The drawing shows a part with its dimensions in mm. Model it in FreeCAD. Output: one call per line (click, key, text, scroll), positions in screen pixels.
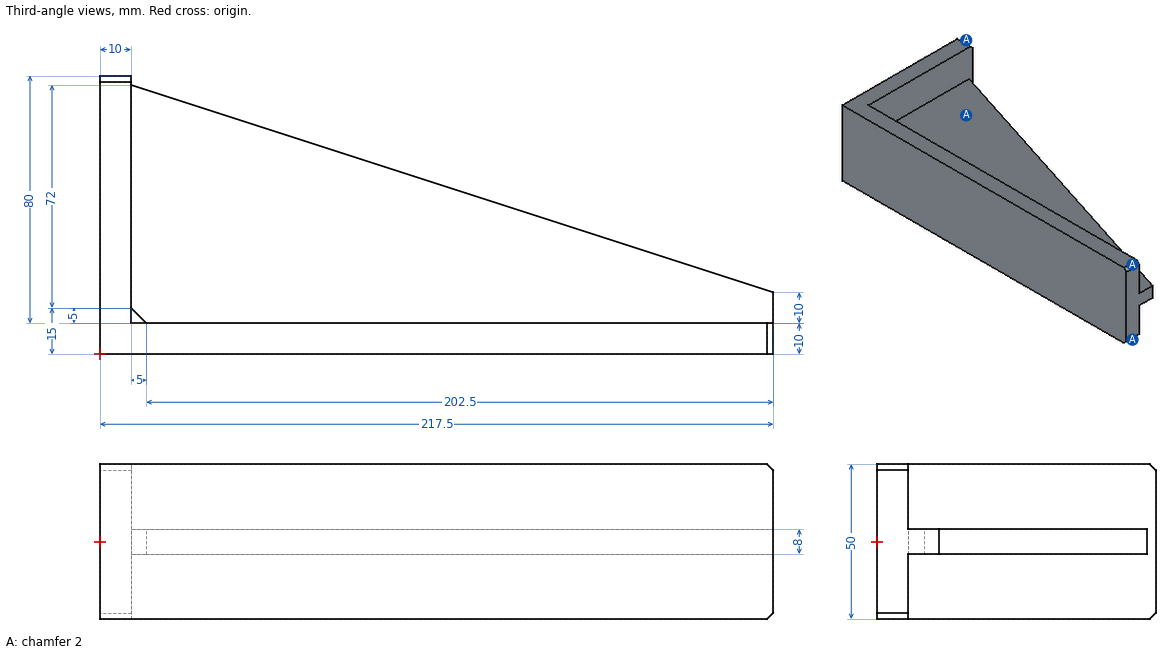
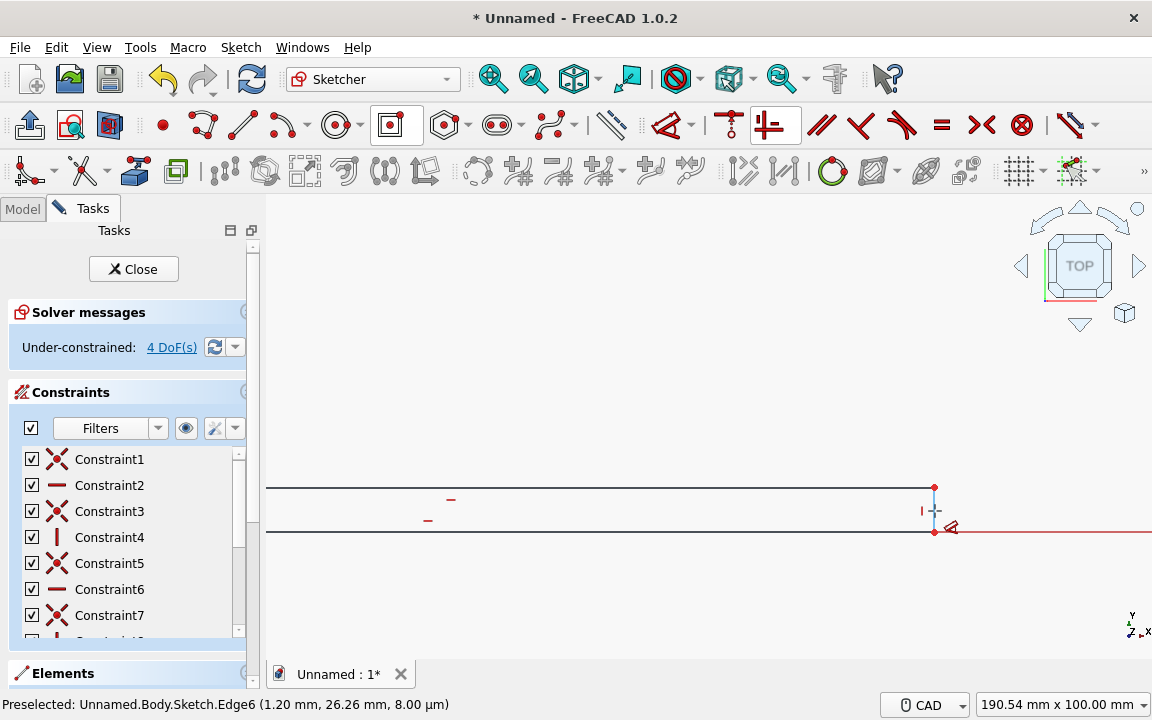
click(934, 510)
click(968, 510)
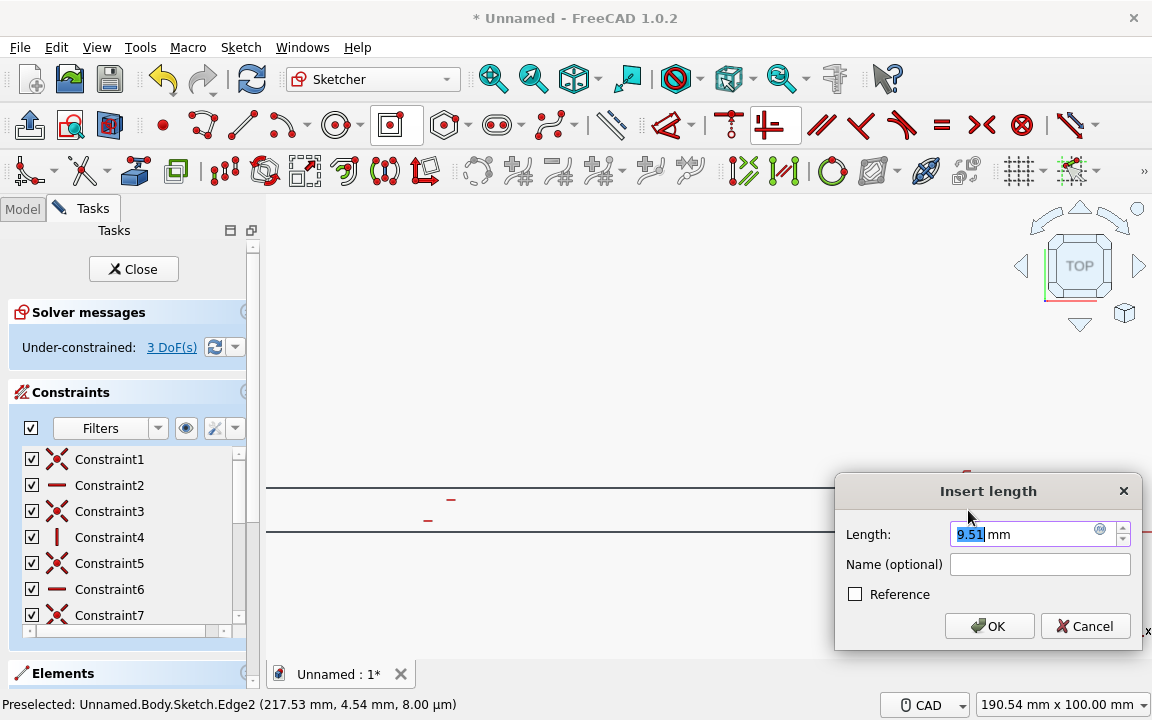
text(10)
key(Return)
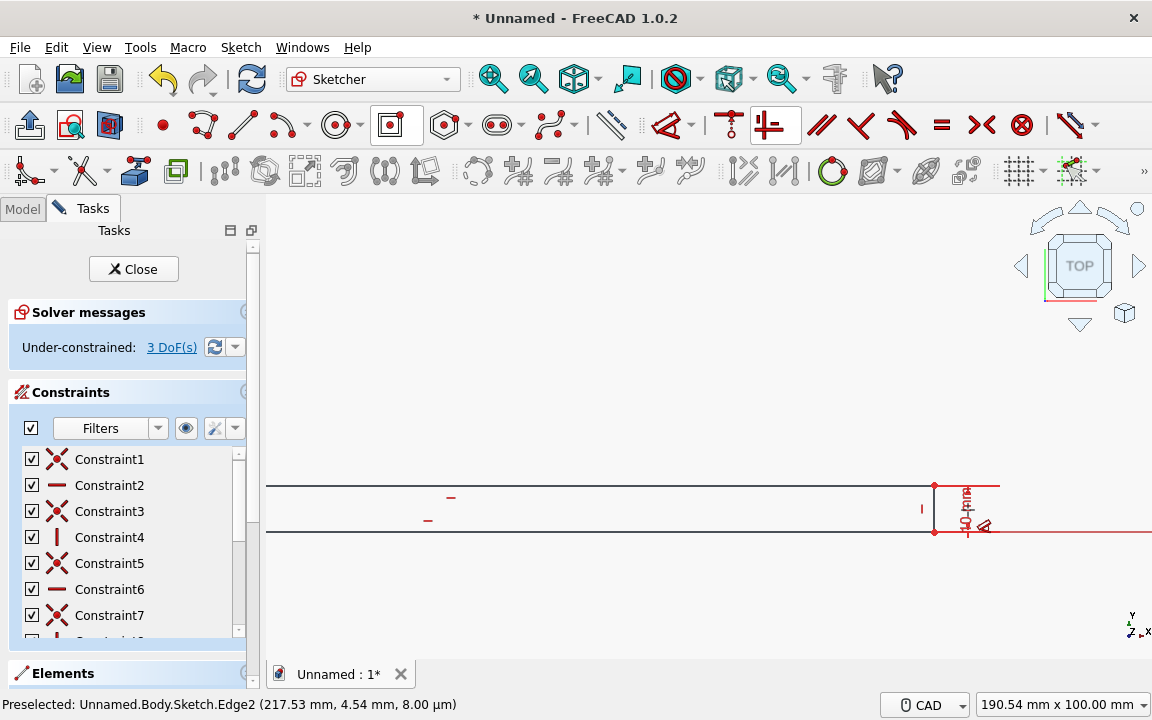
scroll(814, 511, down, 4)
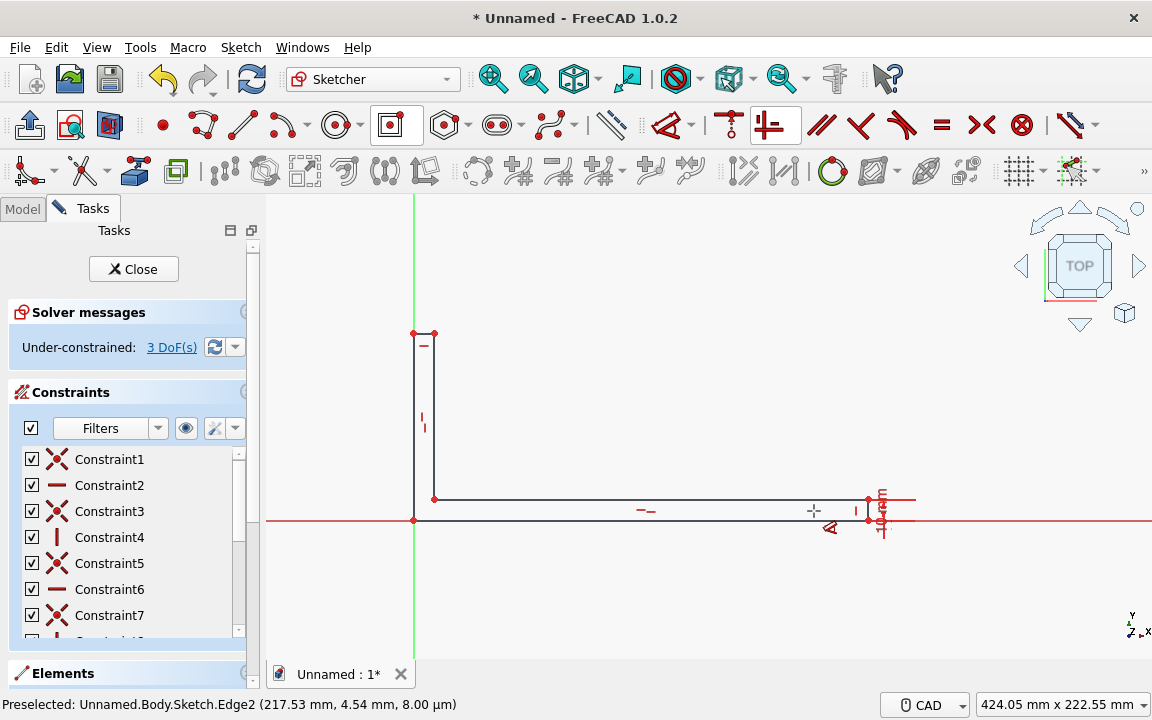
click(434, 450)
click(400, 417)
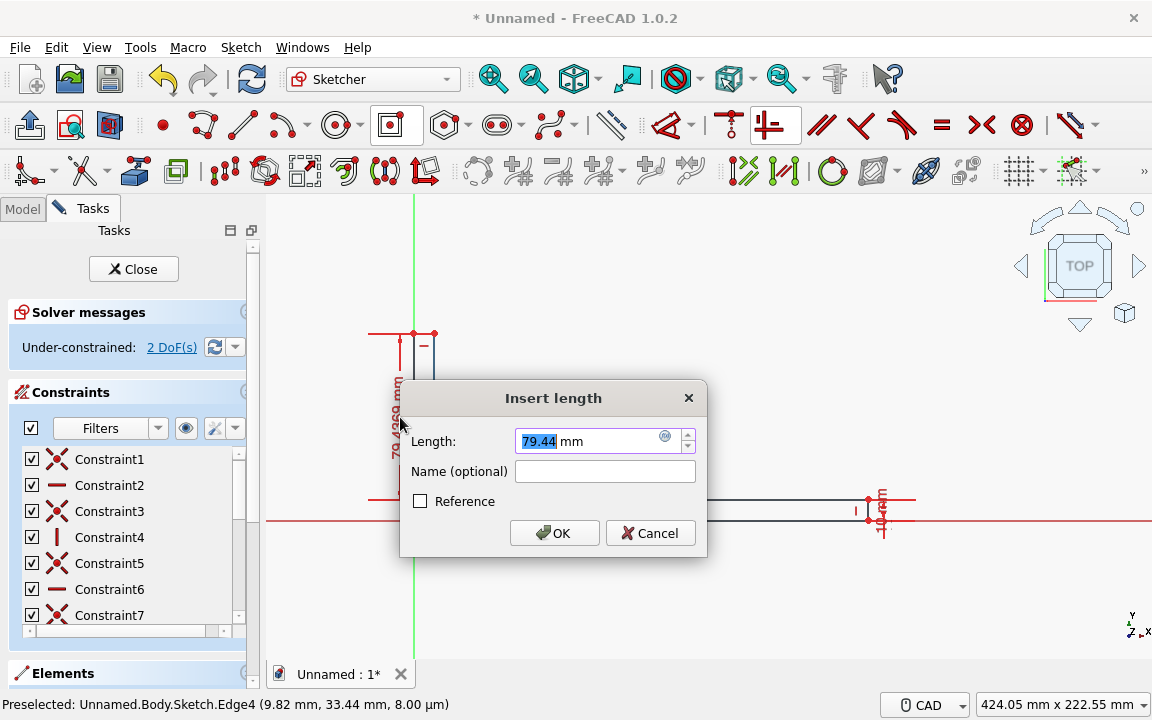
text(80)
key(Return)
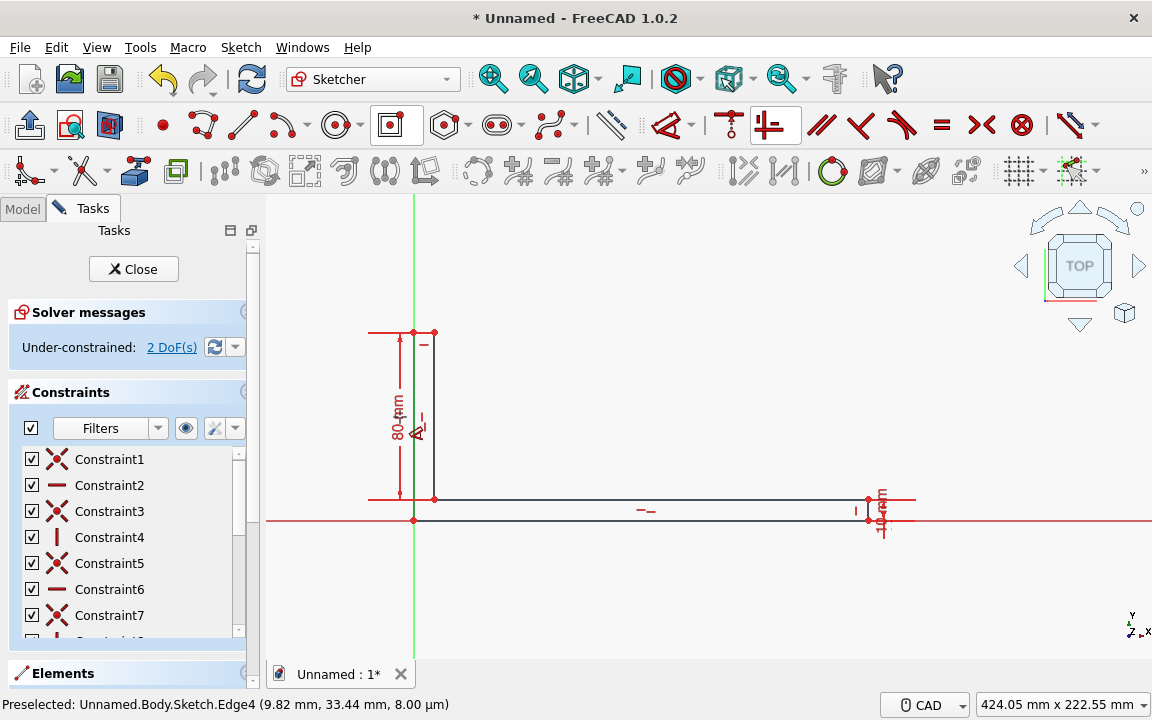
scroll(424, 333, up, 4)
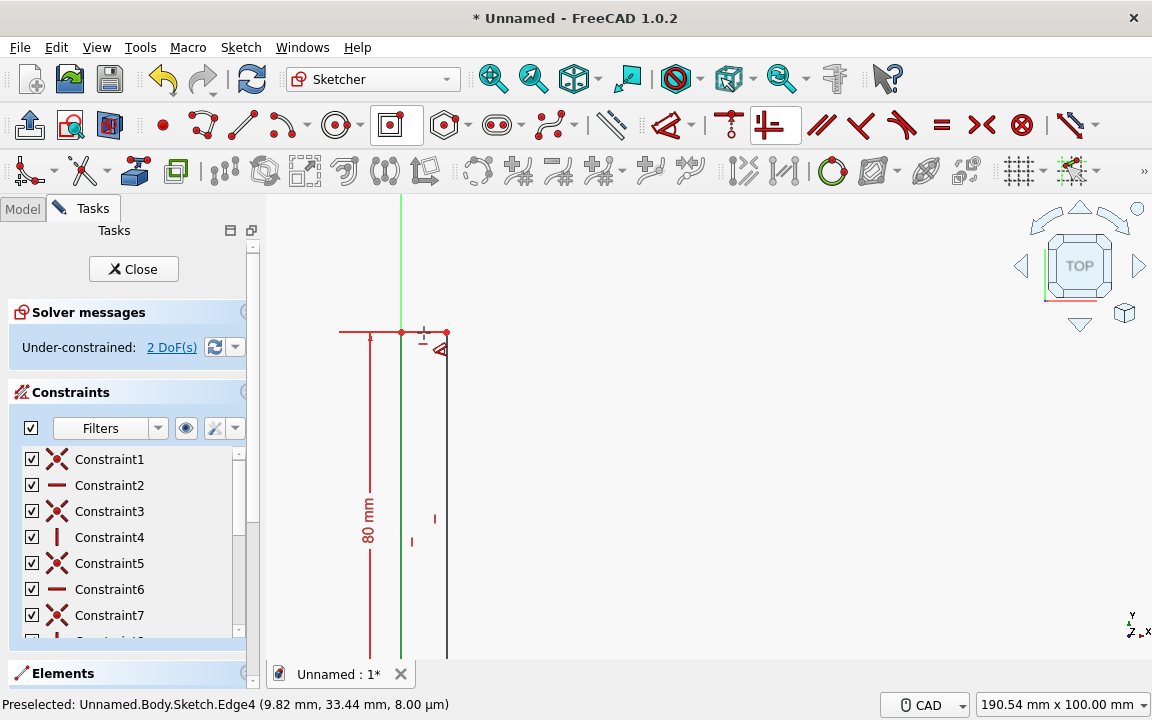
click(424, 332)
click(424, 298)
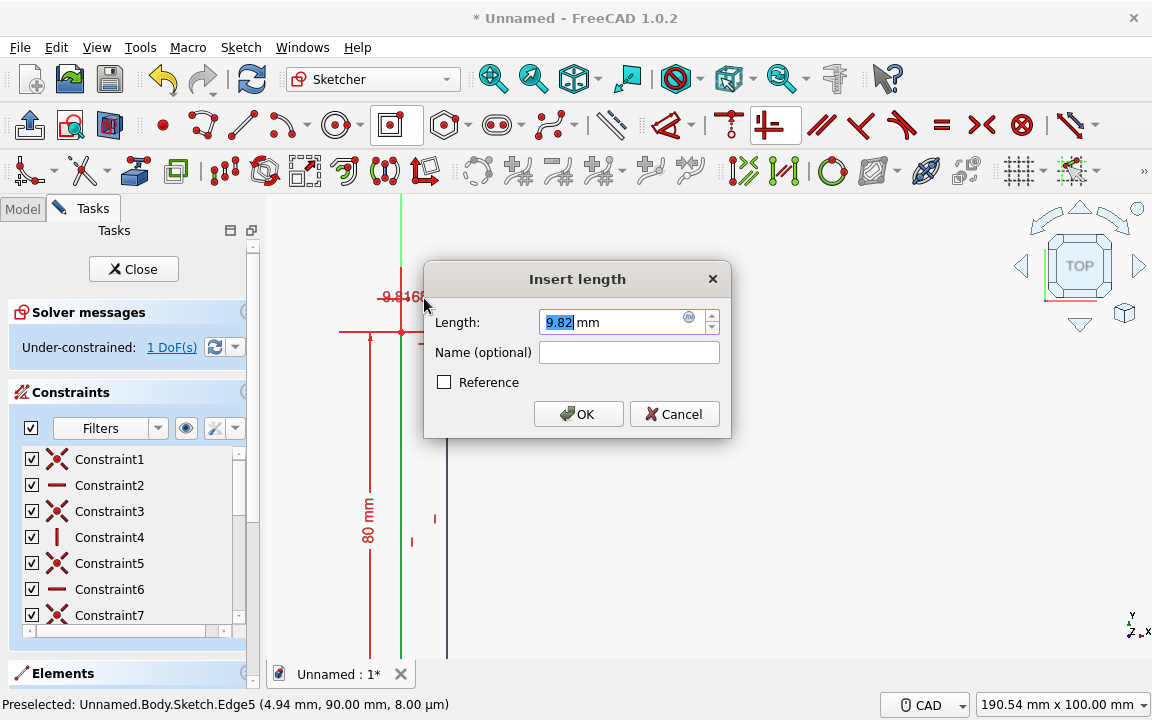
text(10)
key(Return)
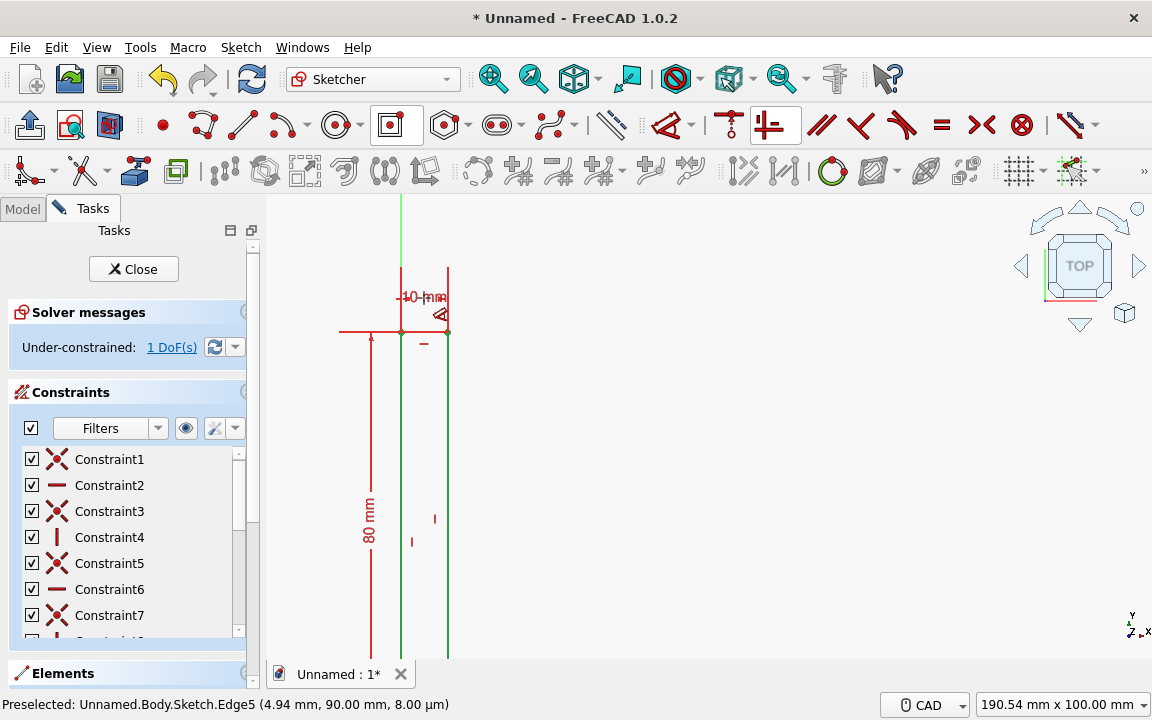
scroll(423, 333, down, 4)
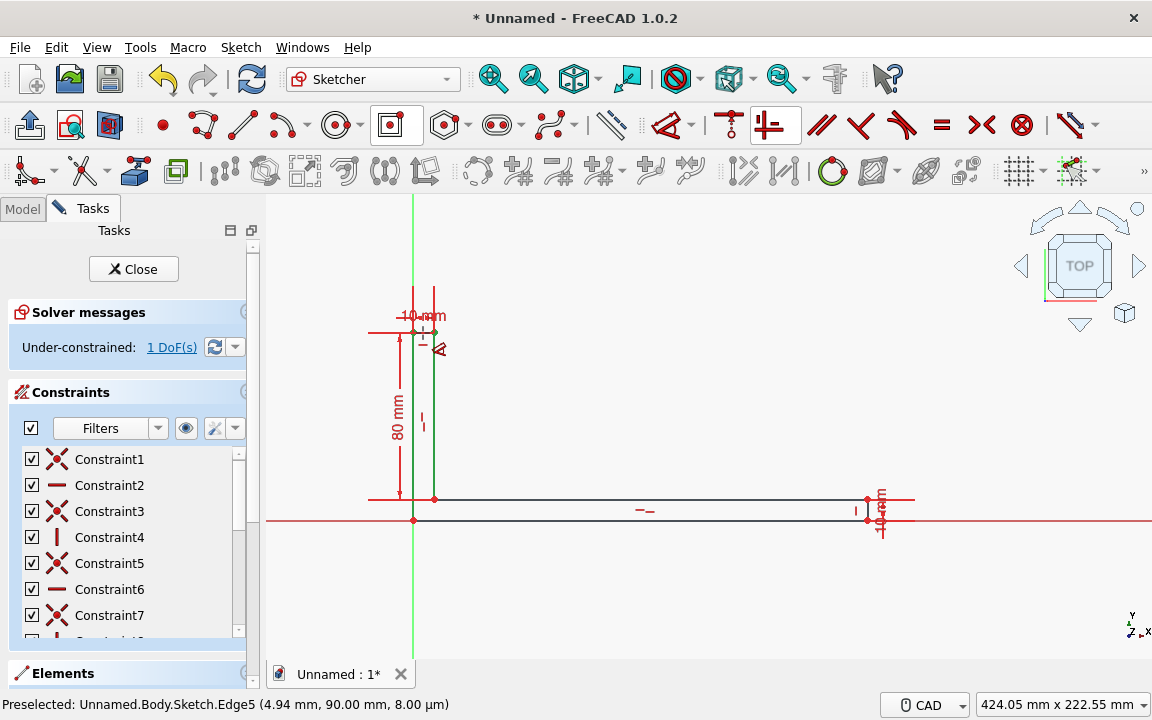
click(550, 521)
click(640, 555)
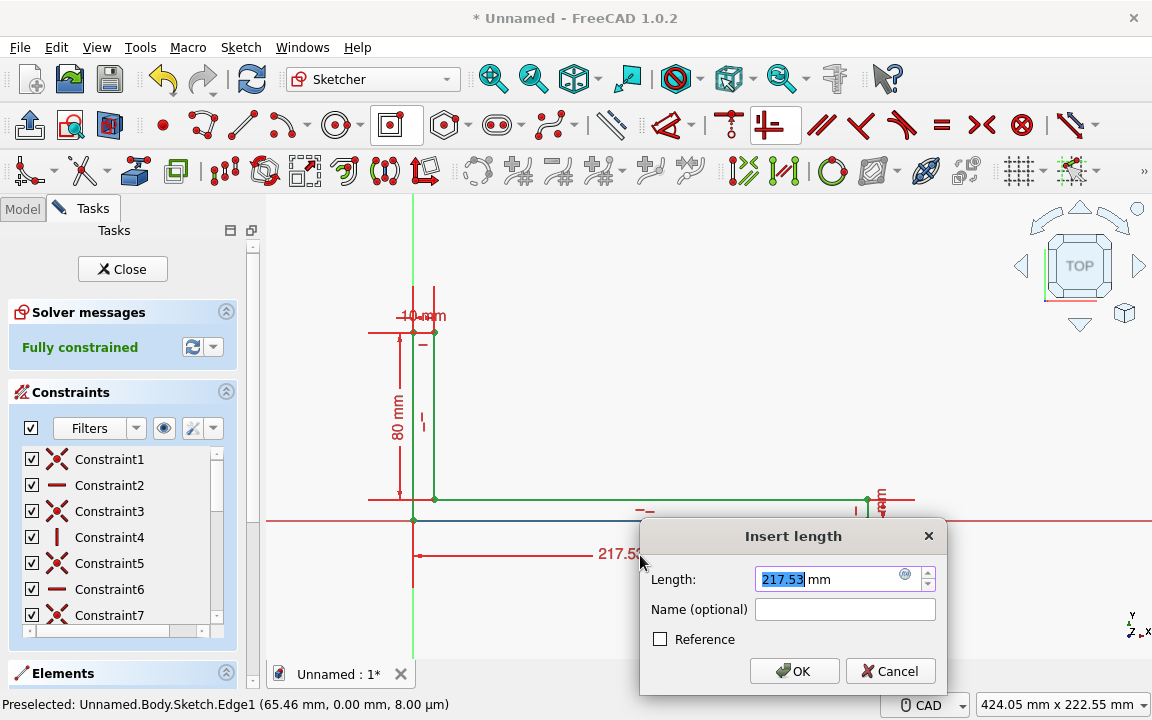
text(217.5)
key(Return)
key(Escape)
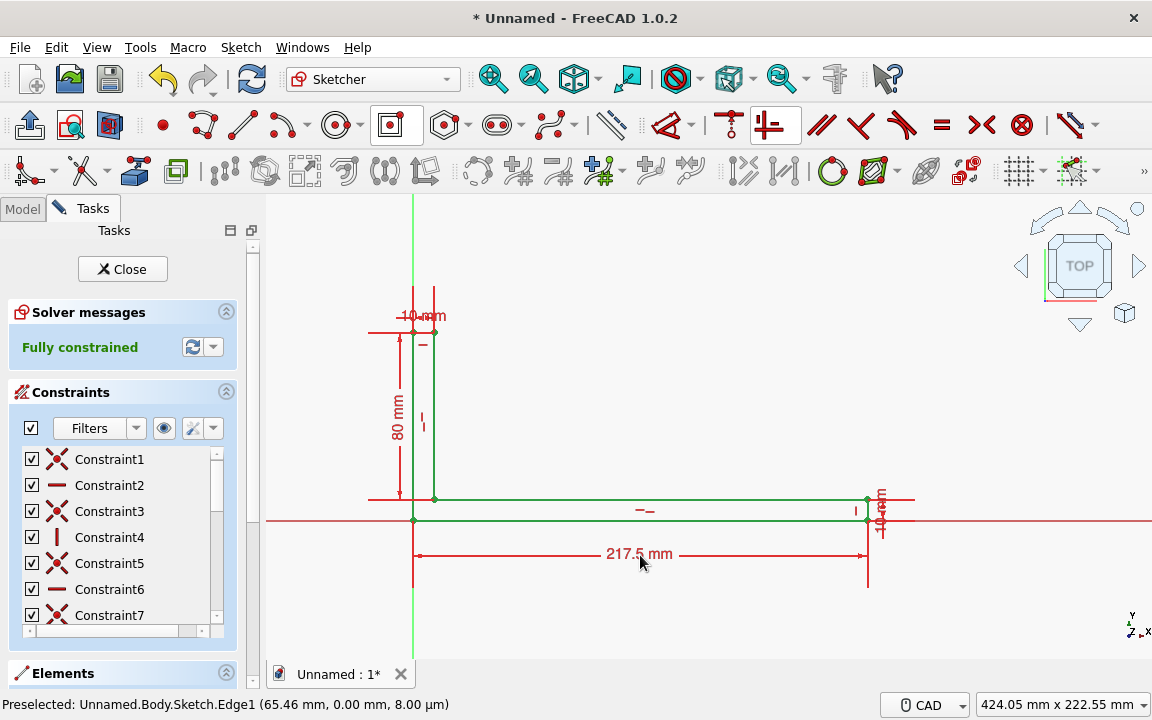
click(123, 269)